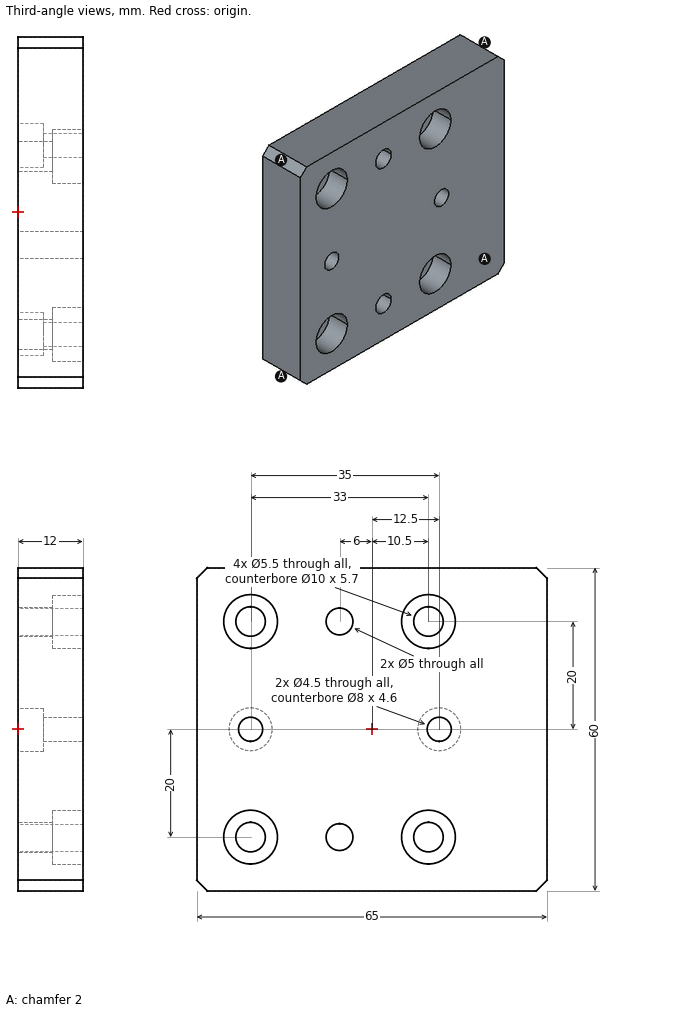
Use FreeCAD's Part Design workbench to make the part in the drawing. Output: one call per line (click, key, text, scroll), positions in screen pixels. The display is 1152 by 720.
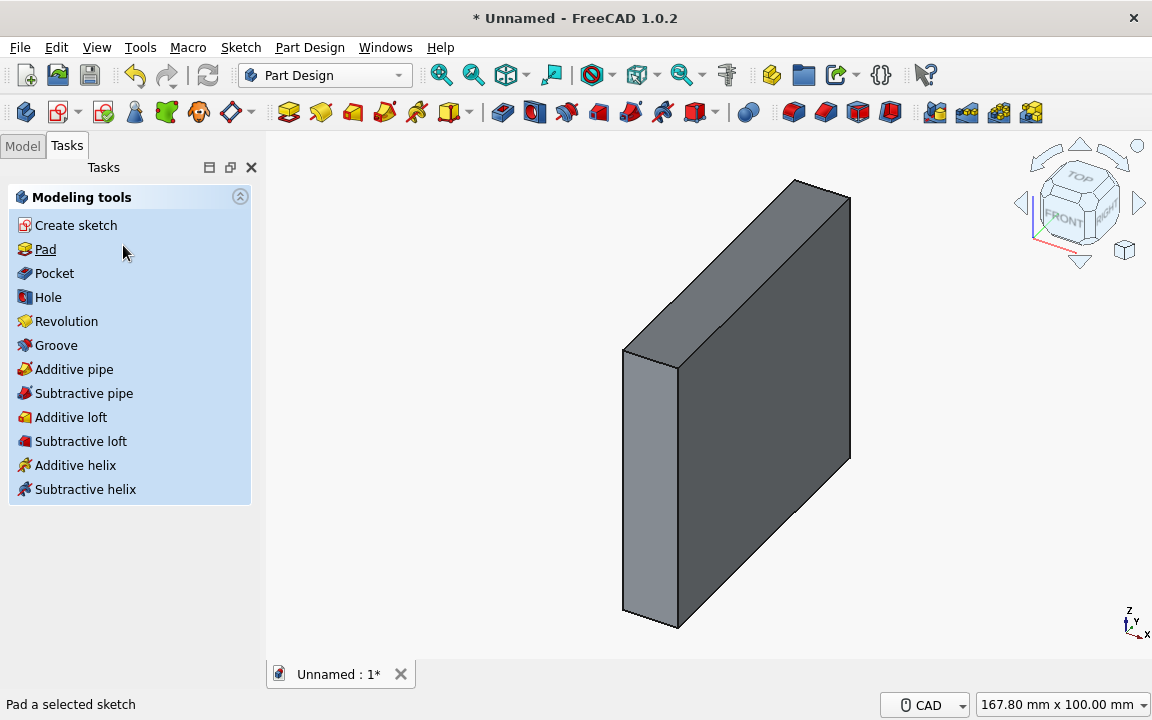
click(536, 112)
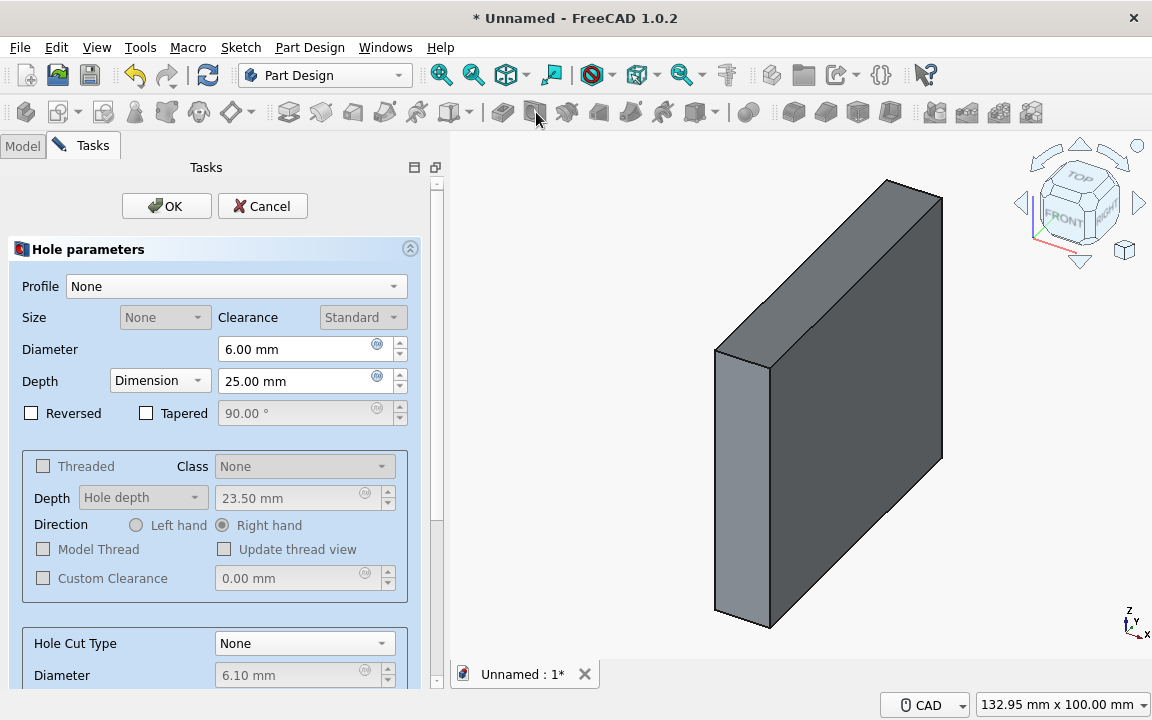
triple_click(305, 349)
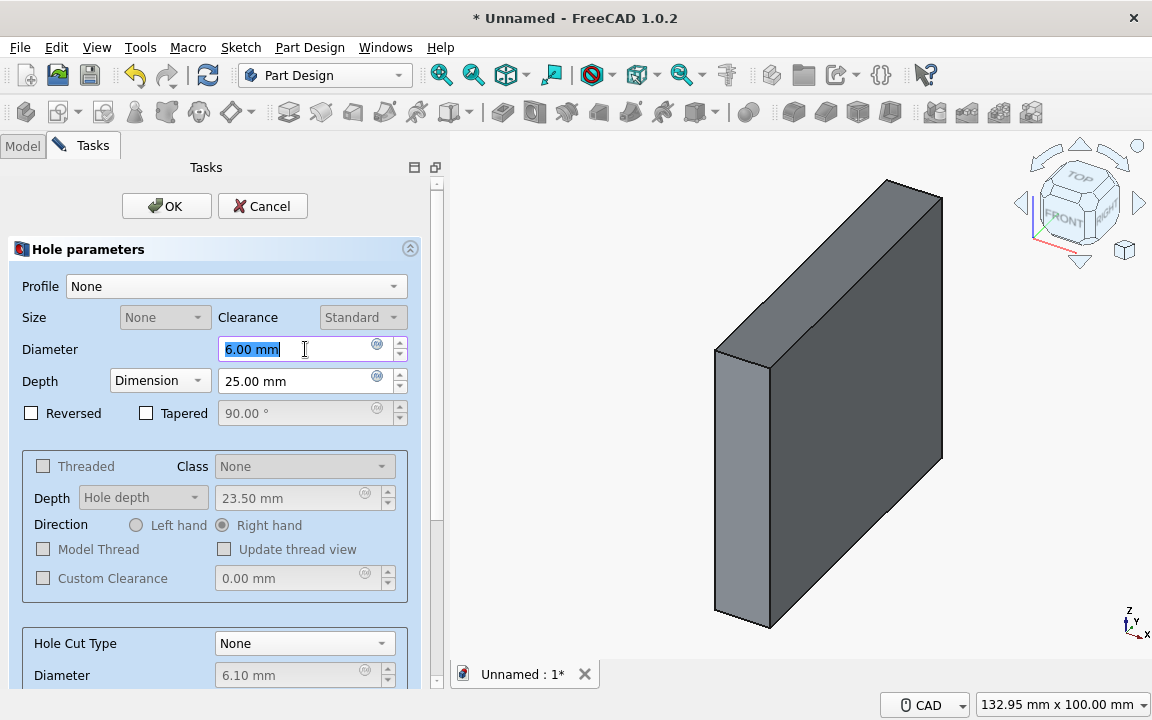
text(4.5)
key(Tab)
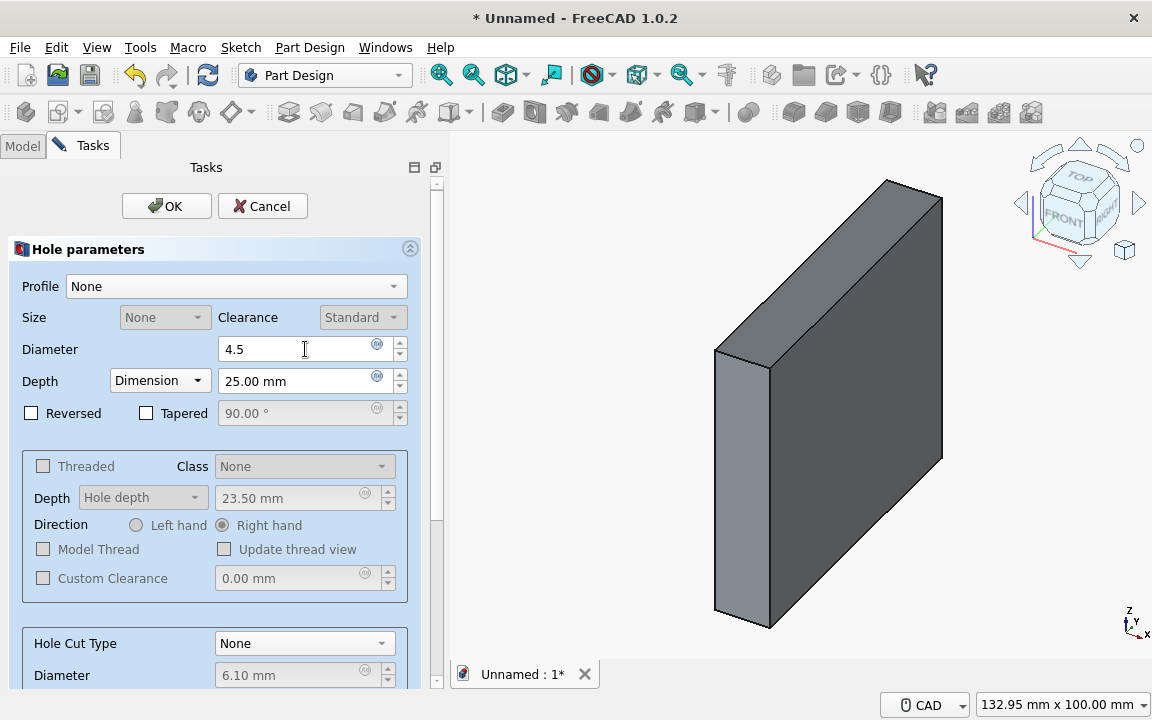
click(161, 380)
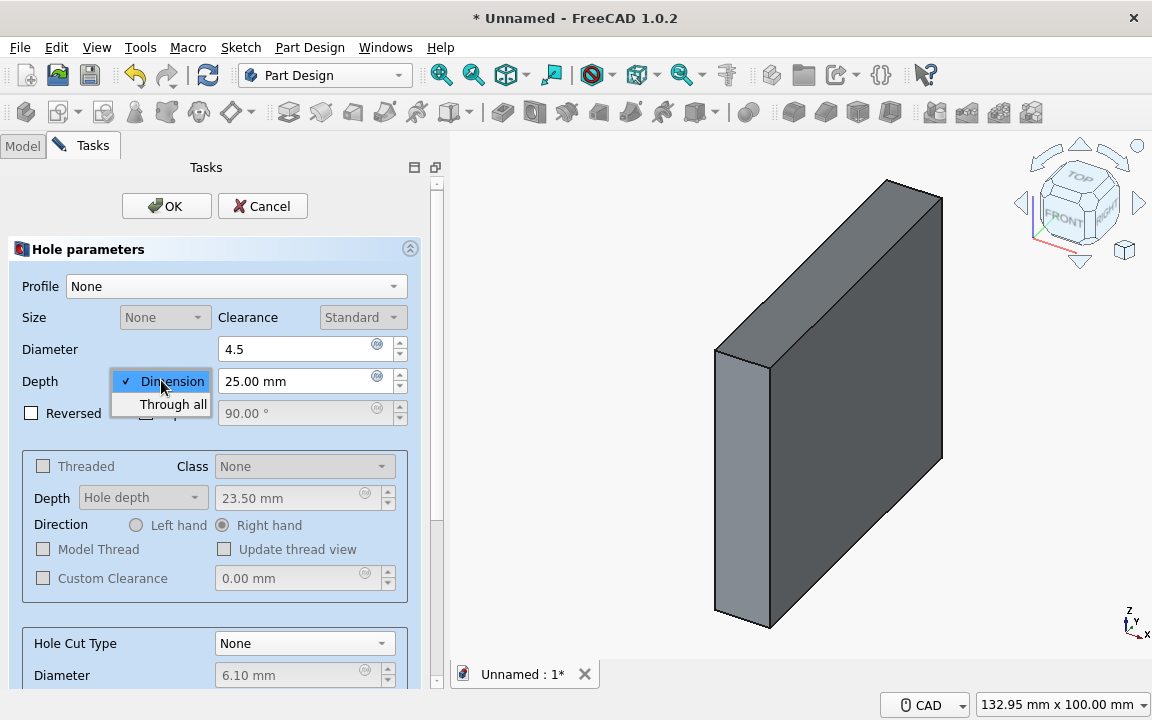
click(160, 404)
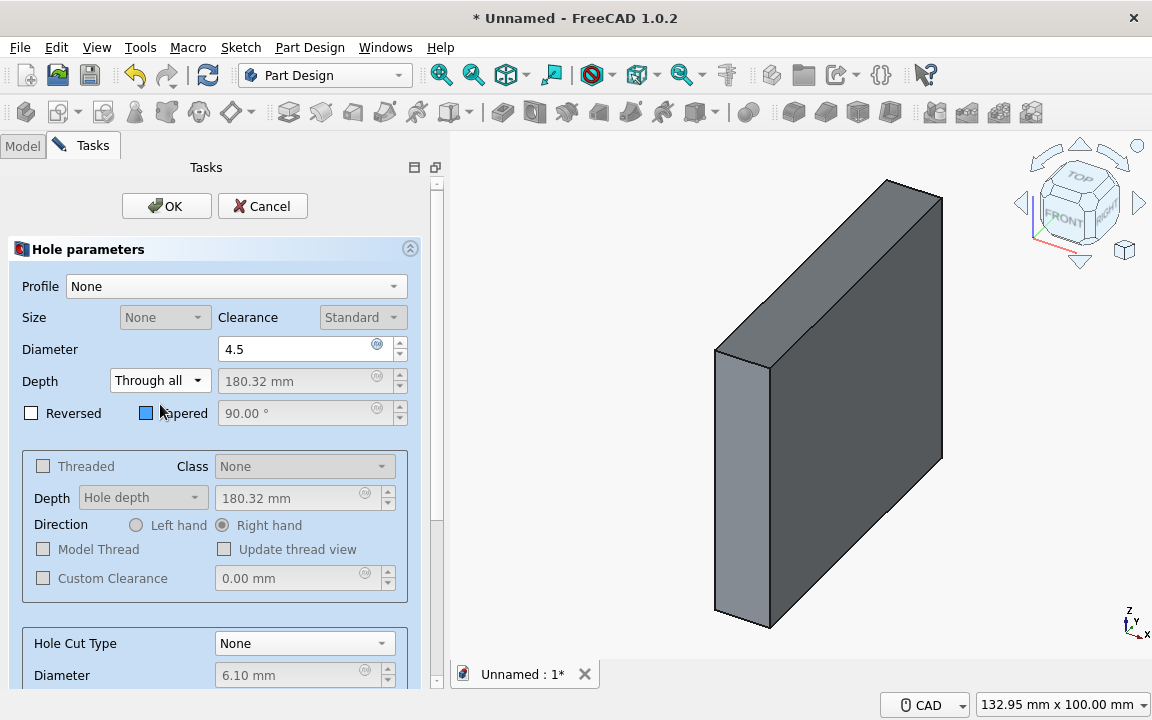
click(30, 413)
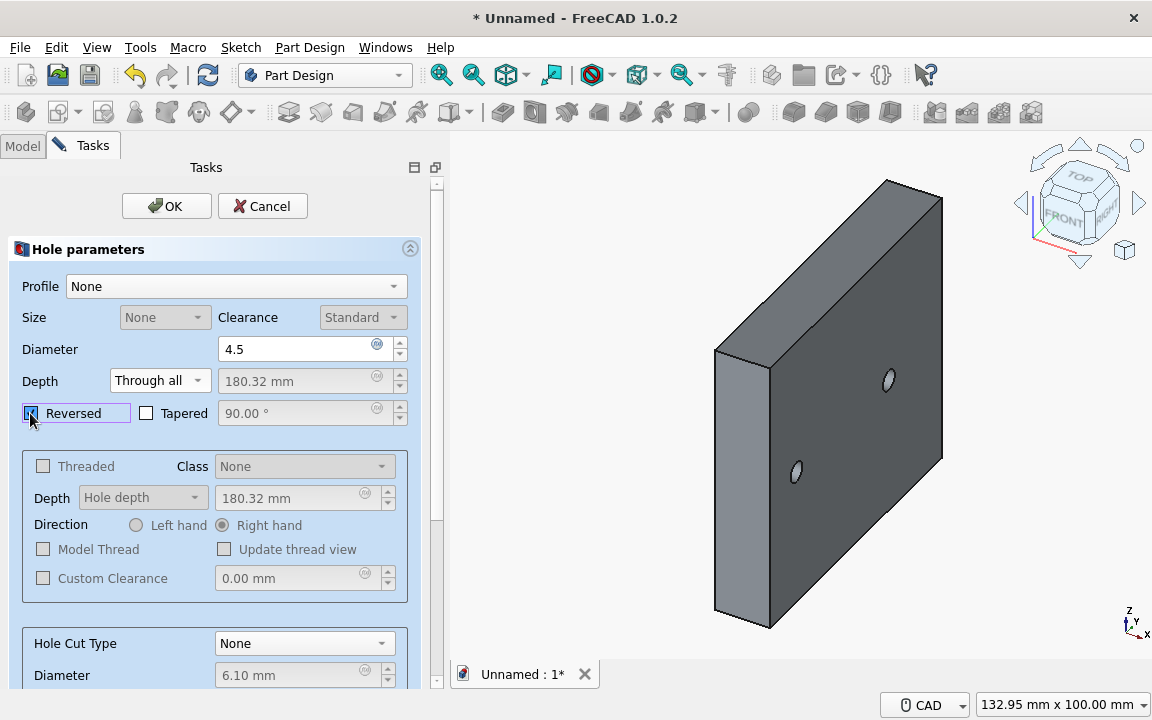
click(306, 644)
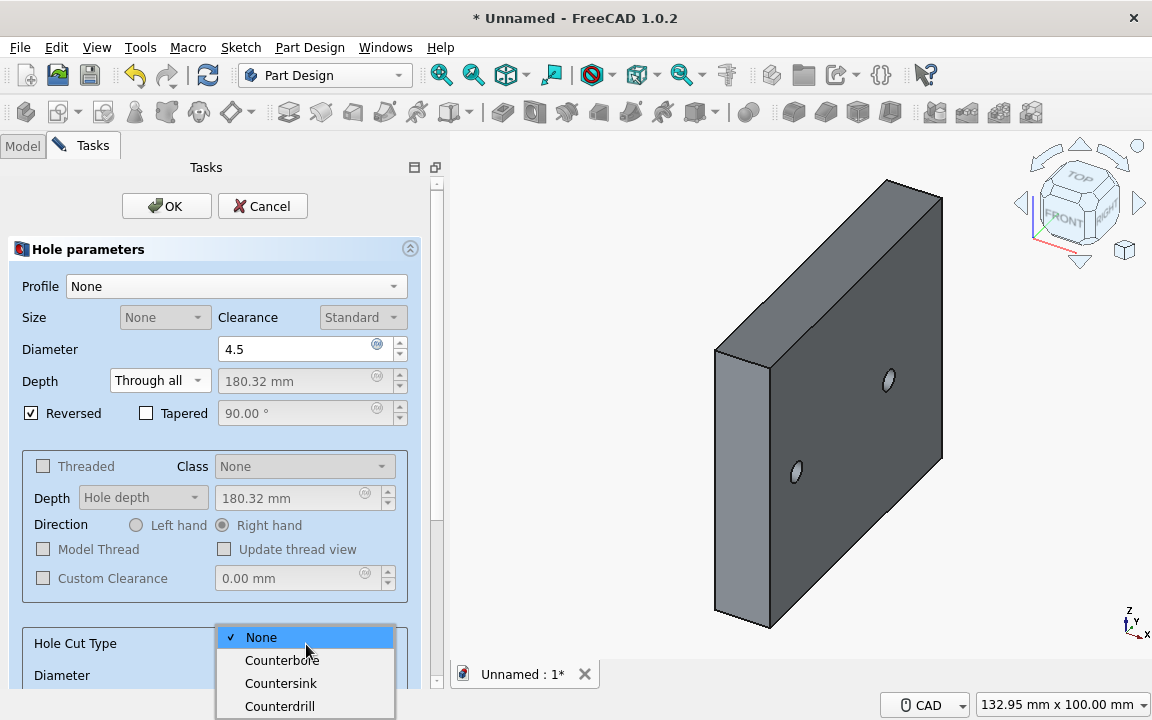
click(304, 660)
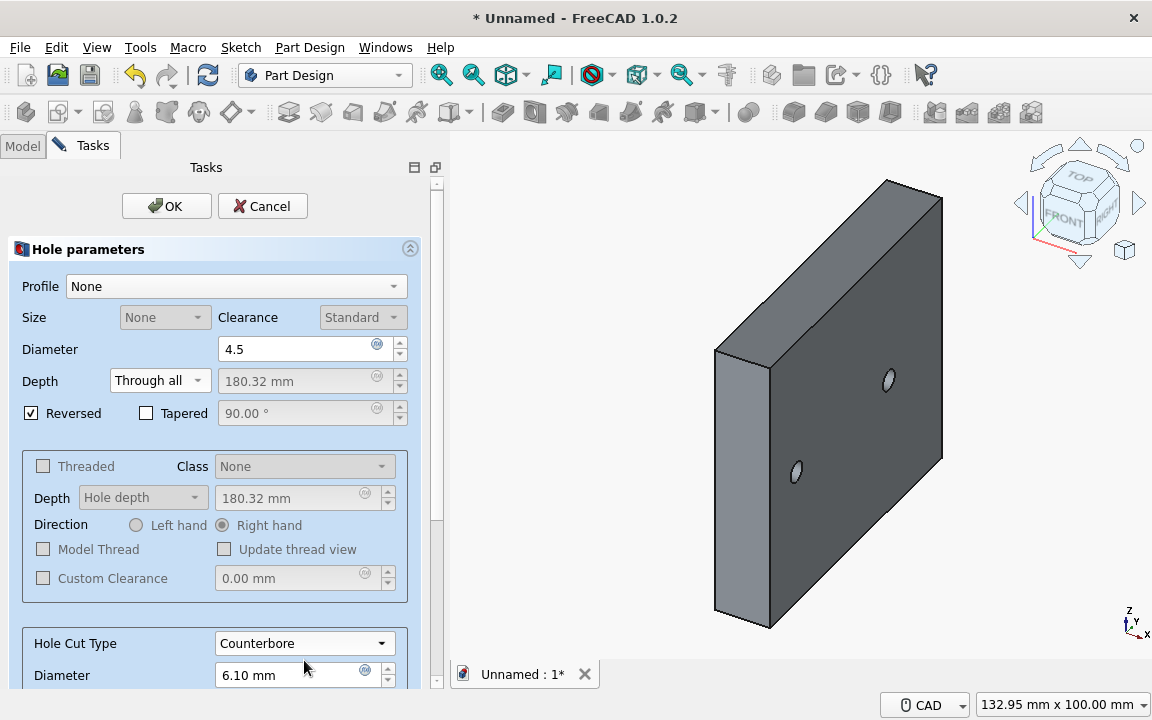
triple_click(298, 675)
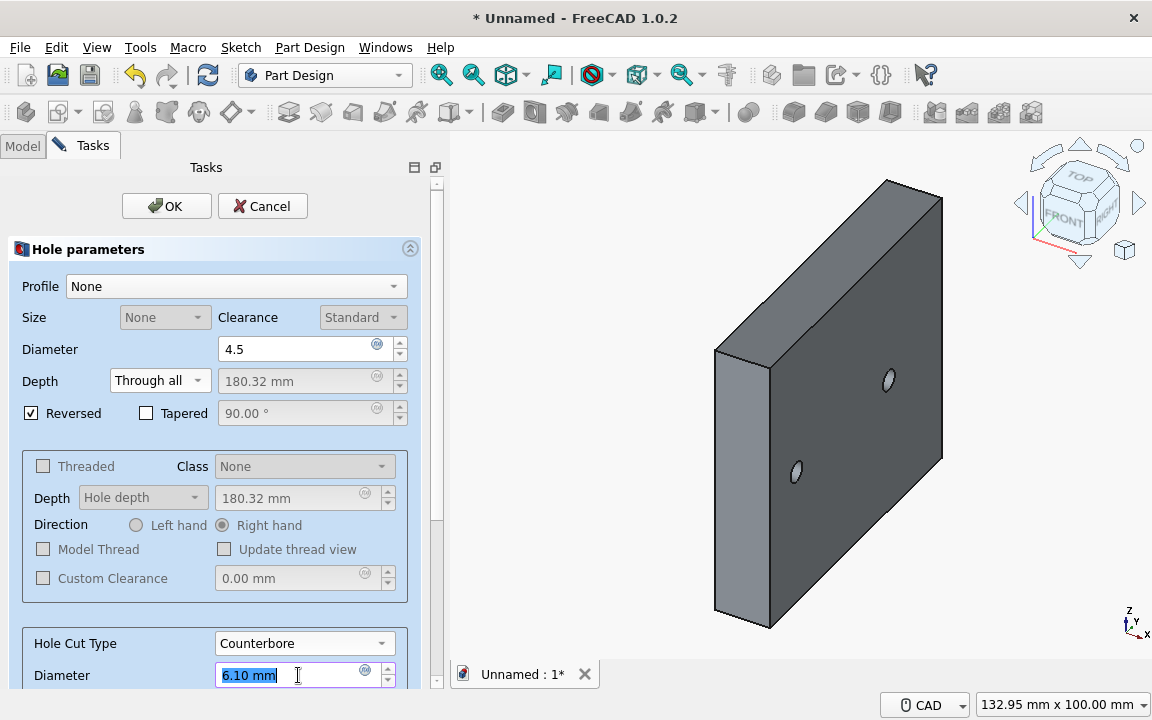
text(8)
key(Tab)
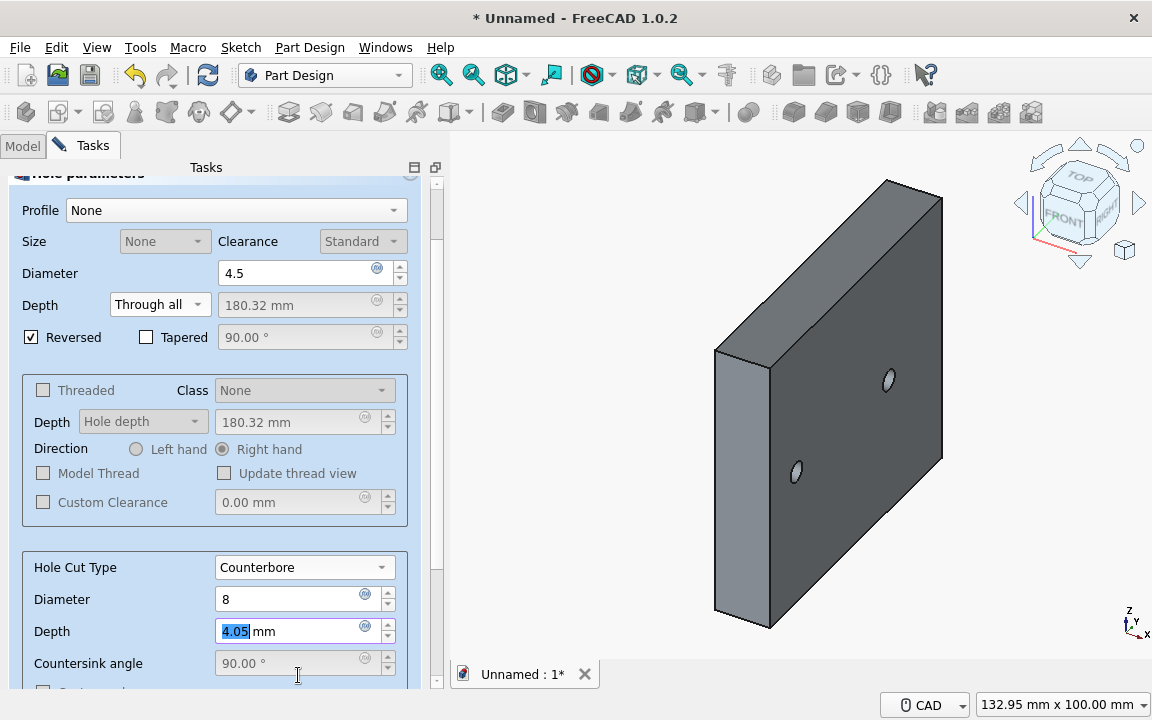
text(4.6)
key(Tab)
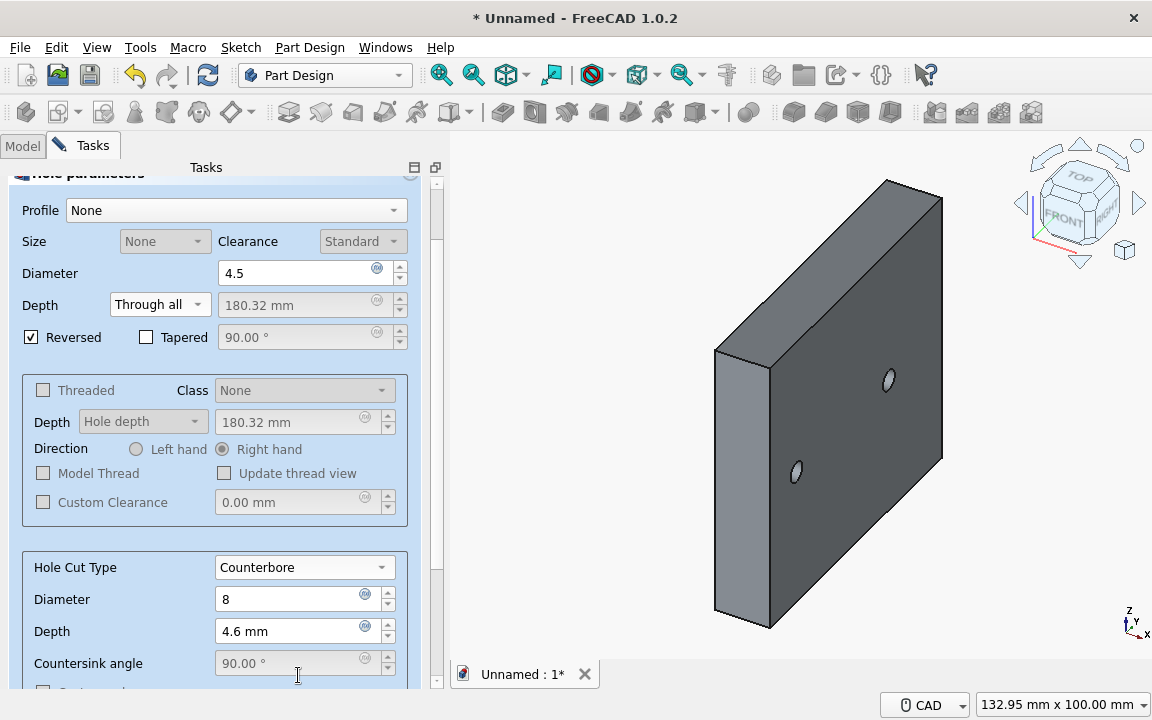
scroll(437, 432, up, 3)